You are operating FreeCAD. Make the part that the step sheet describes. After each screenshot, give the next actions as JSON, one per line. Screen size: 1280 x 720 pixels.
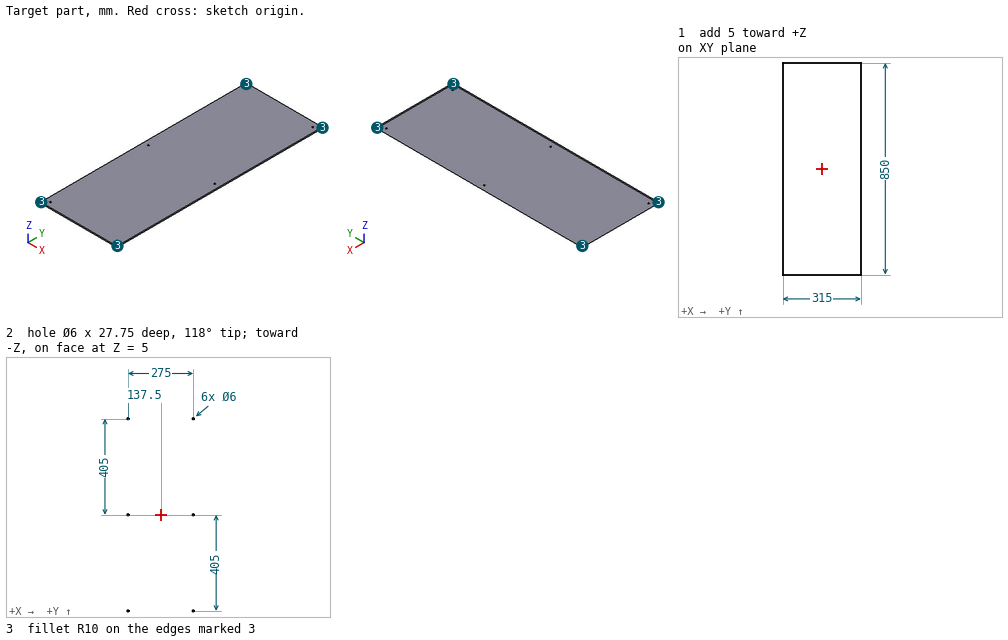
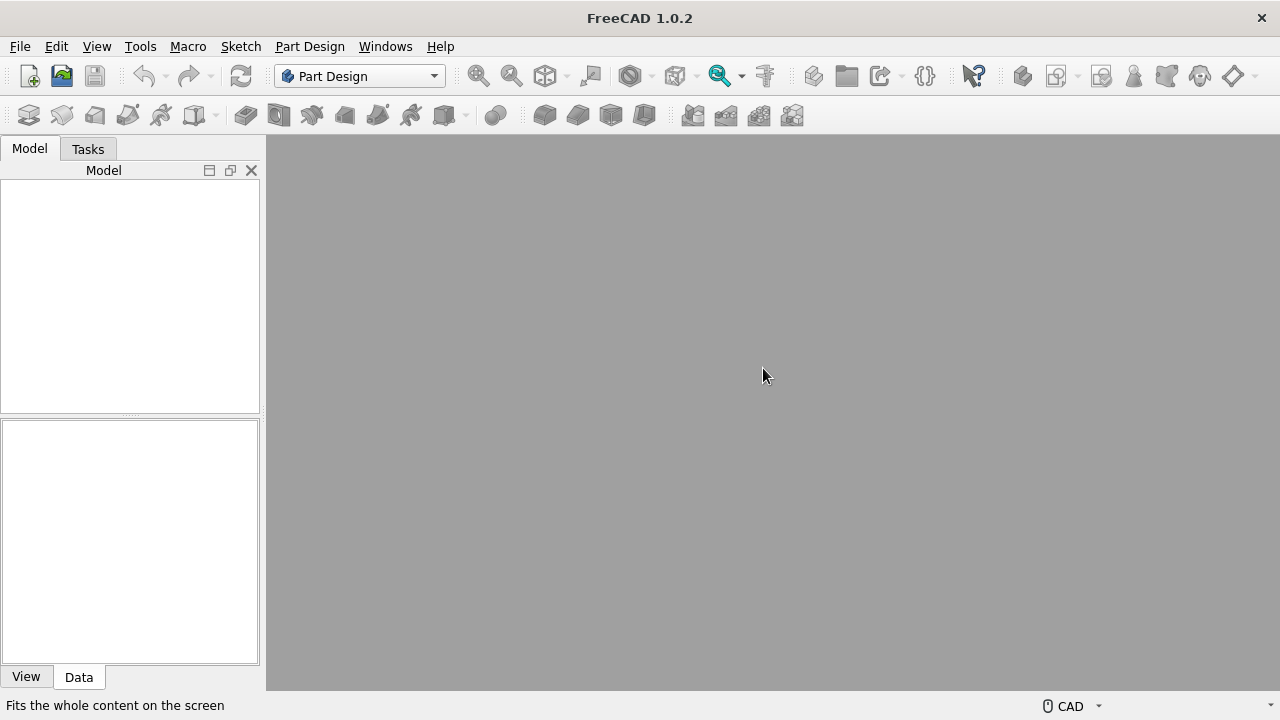
{"action": "left_click", "coordinate": [29, 76]}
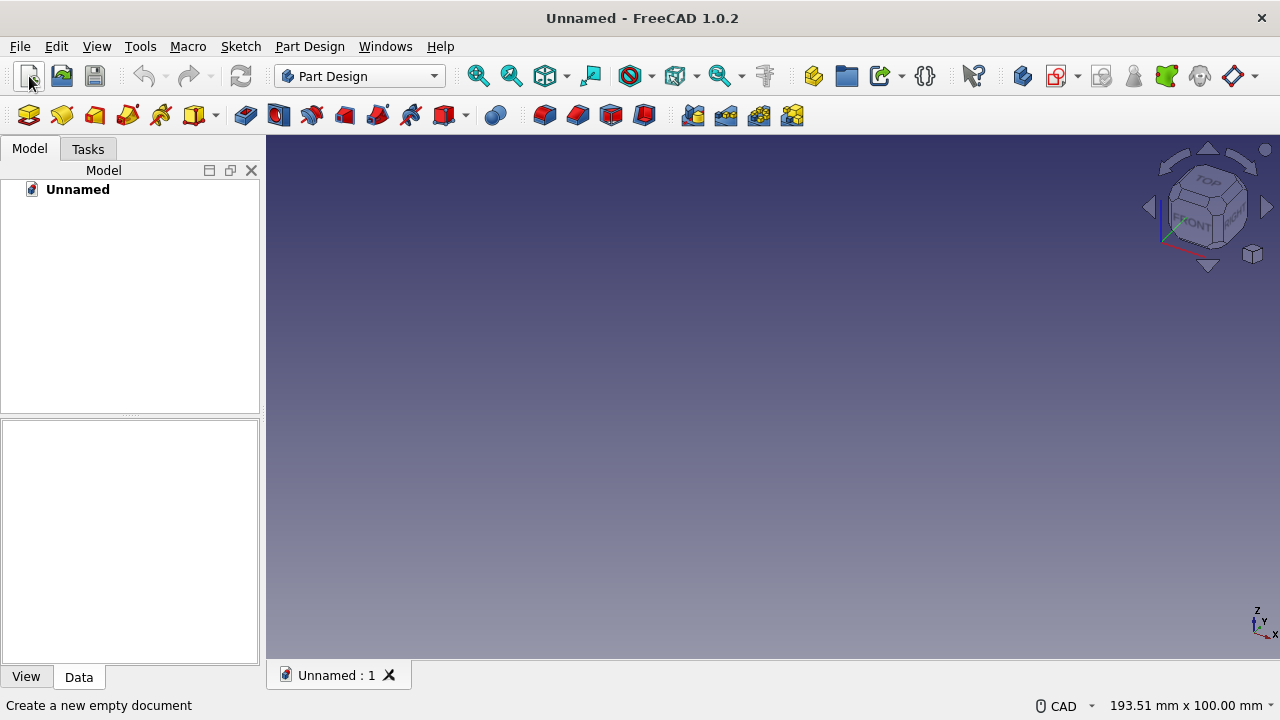
{"action": "left_click", "coordinate": [1056, 76]}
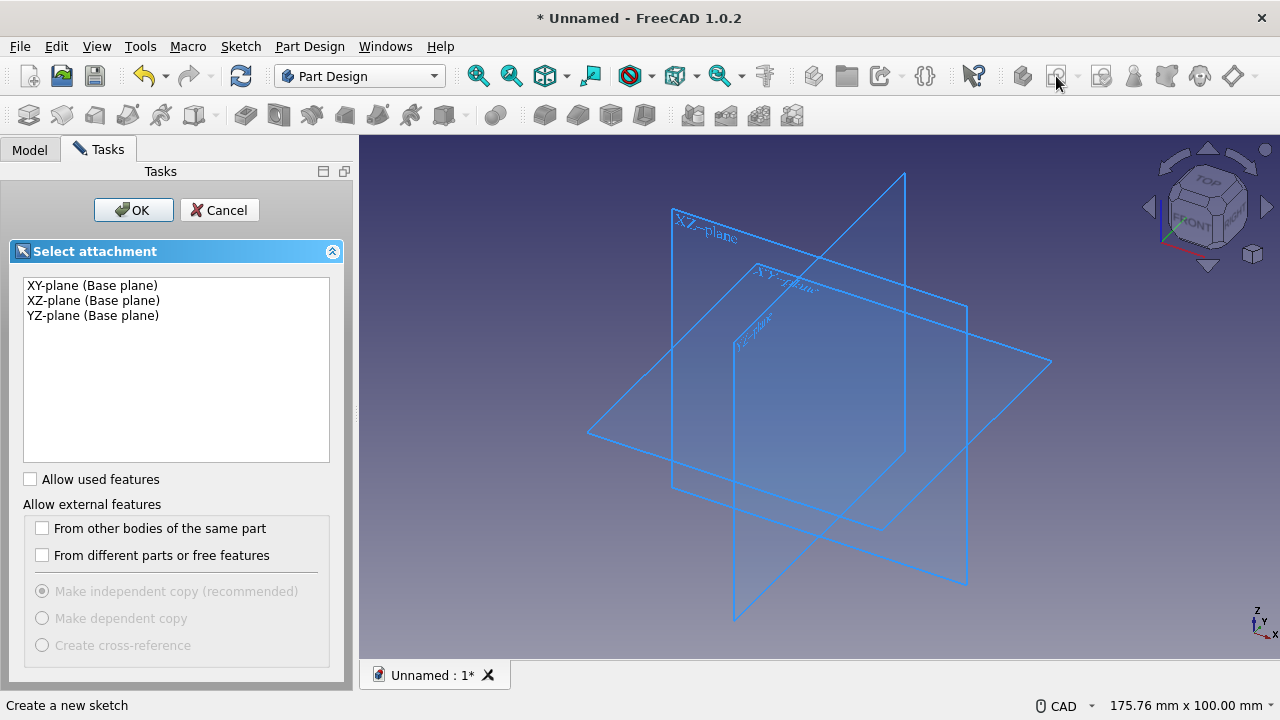
{"action": "left_click", "coordinate": [84, 286]}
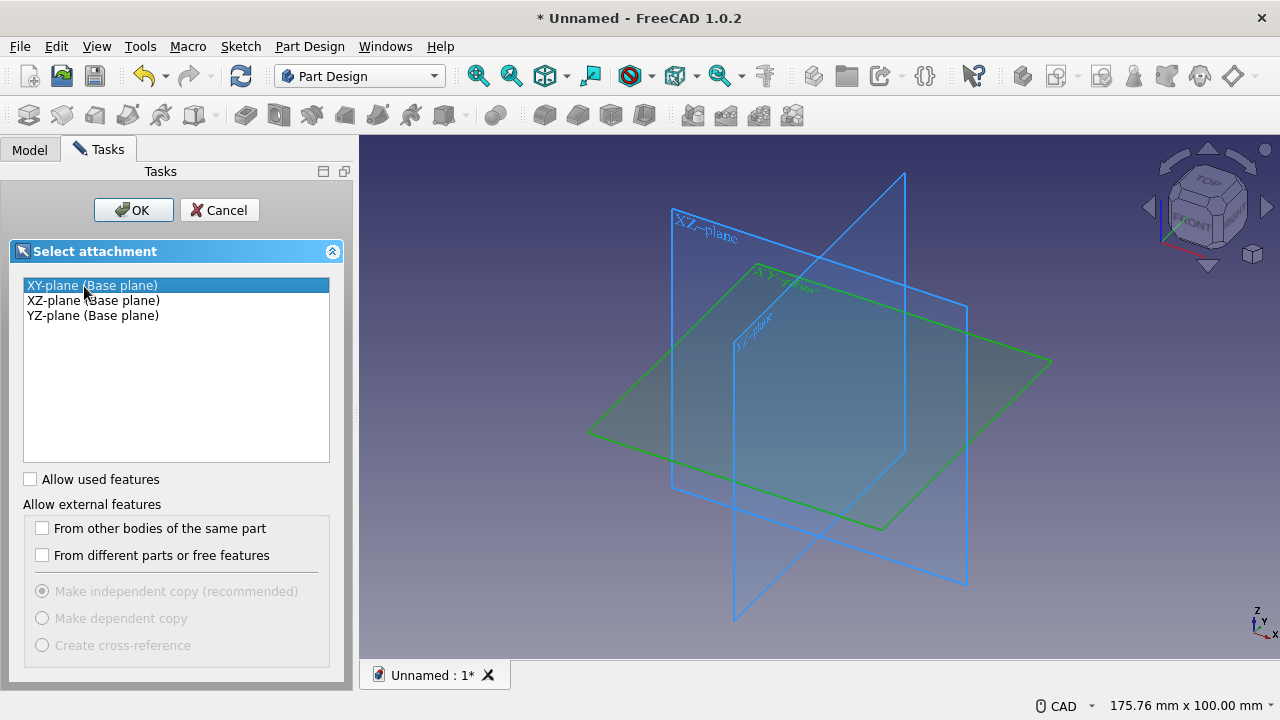
{"action": "left_click", "coordinate": [134, 210]}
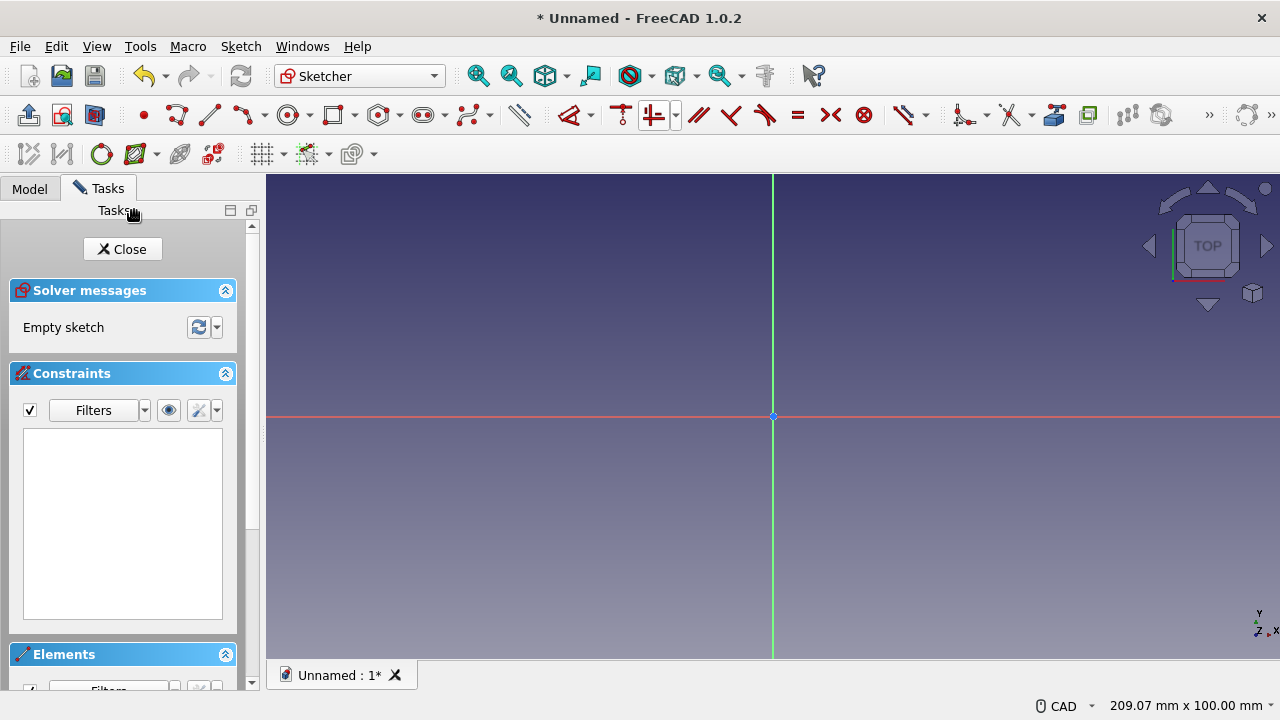
{"action": "scroll", "coordinate": [699, 416], "scroll_direction": "down", "scroll_amount": 13}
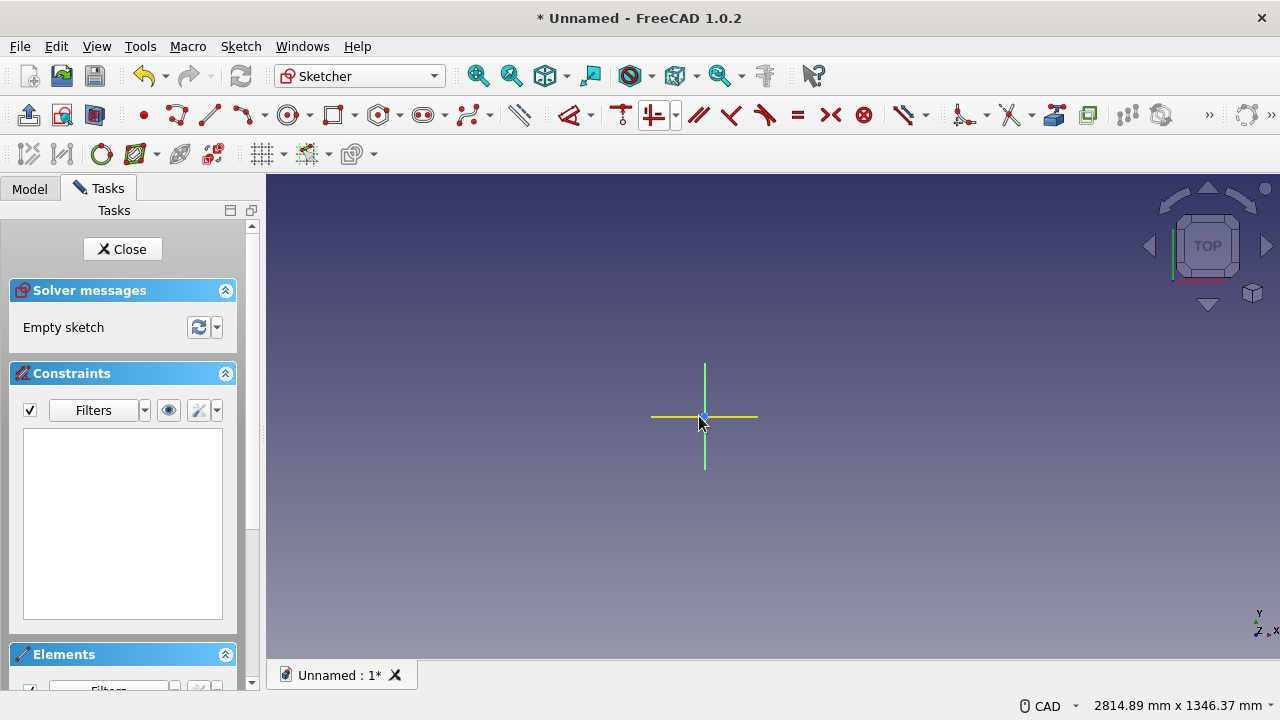
{"action": "left_click", "coordinate": [354, 116]}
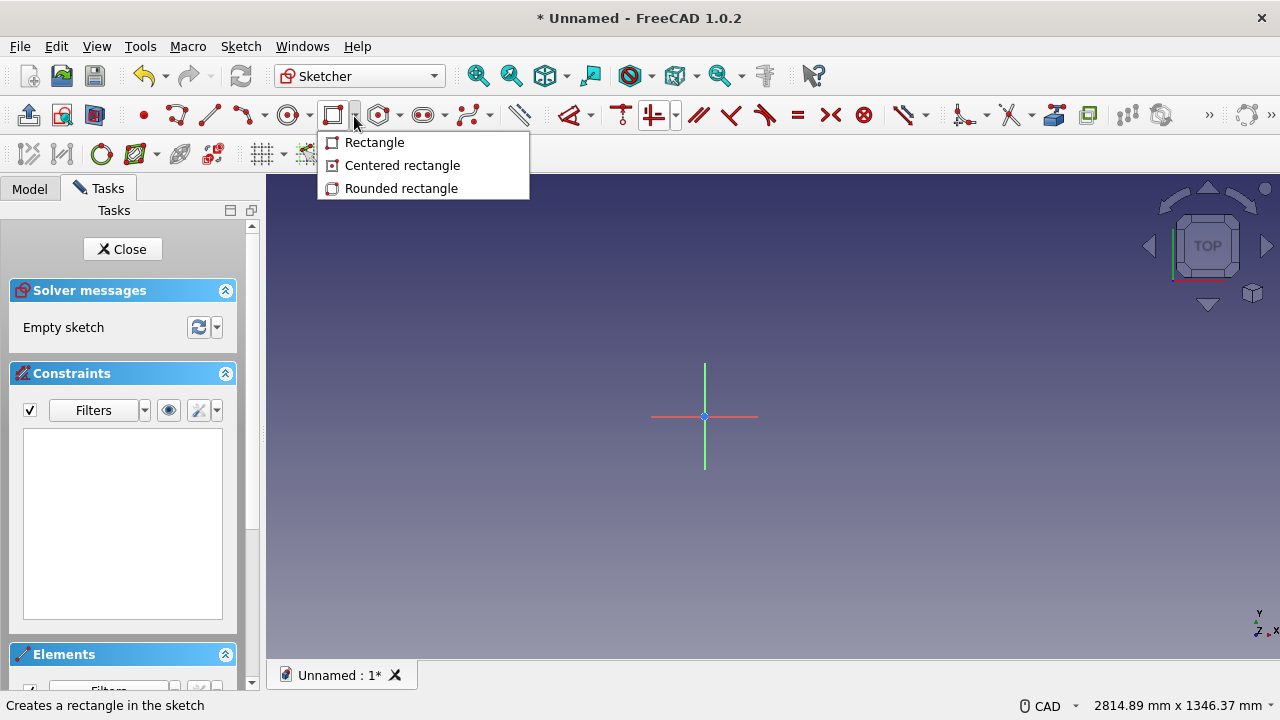
{"action": "left_click", "coordinate": [424, 166]}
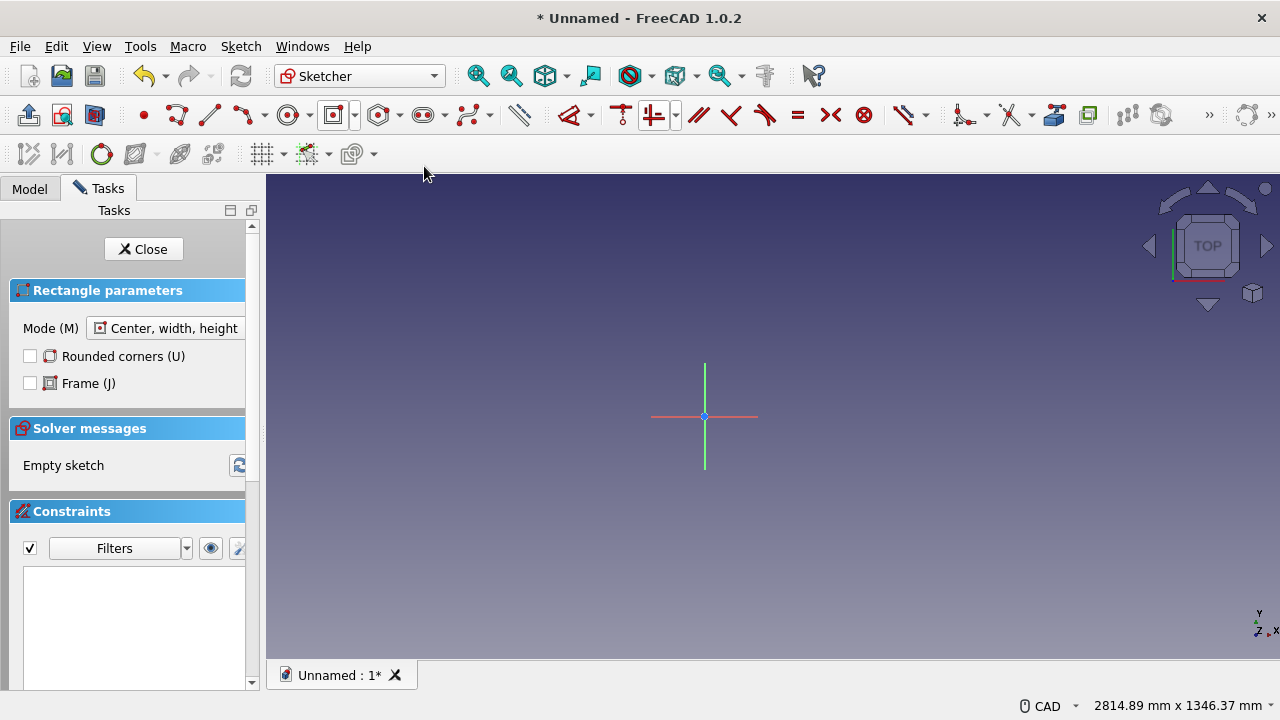
{"action": "left_click", "coordinate": [705, 416]}
{"action": "mouse_move", "coordinate": [762, 263]}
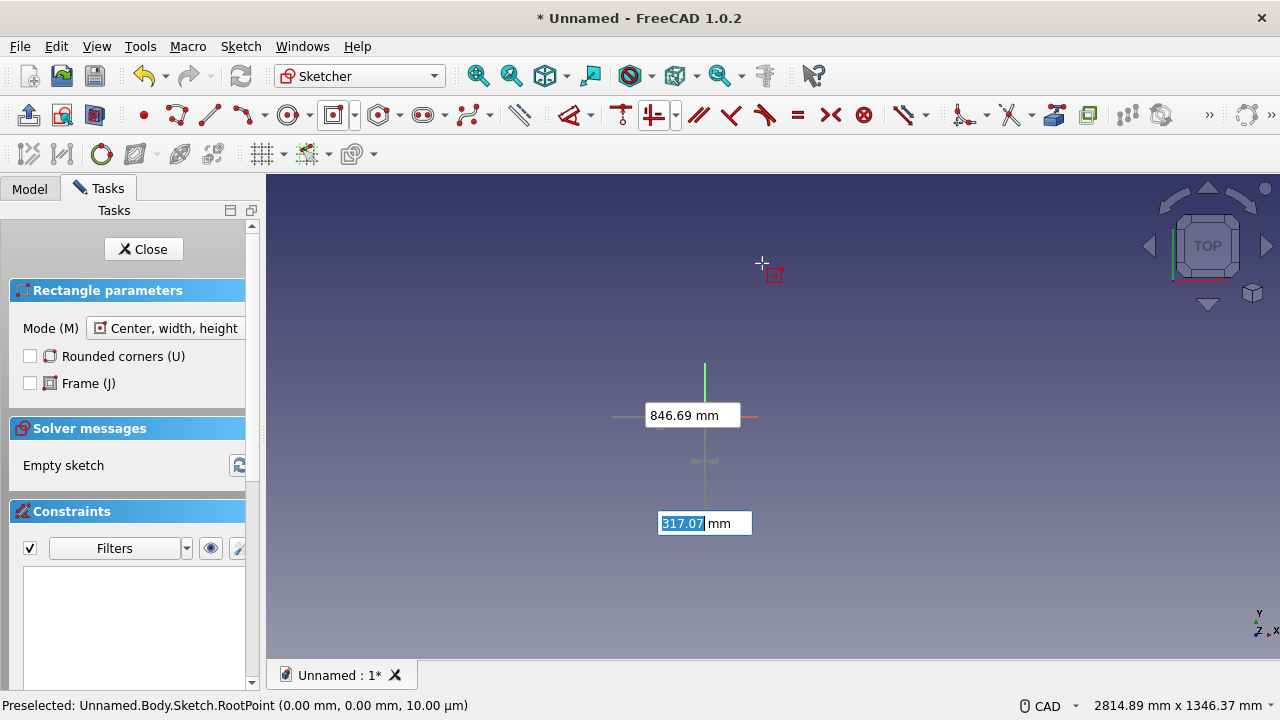
{"action": "type", "text": "315"}
{"action": "key", "text": "Tab"}
{"action": "type", "text": "850"}
{"action": "key", "text": "Return"}
{"action": "key", "text": "Escape"}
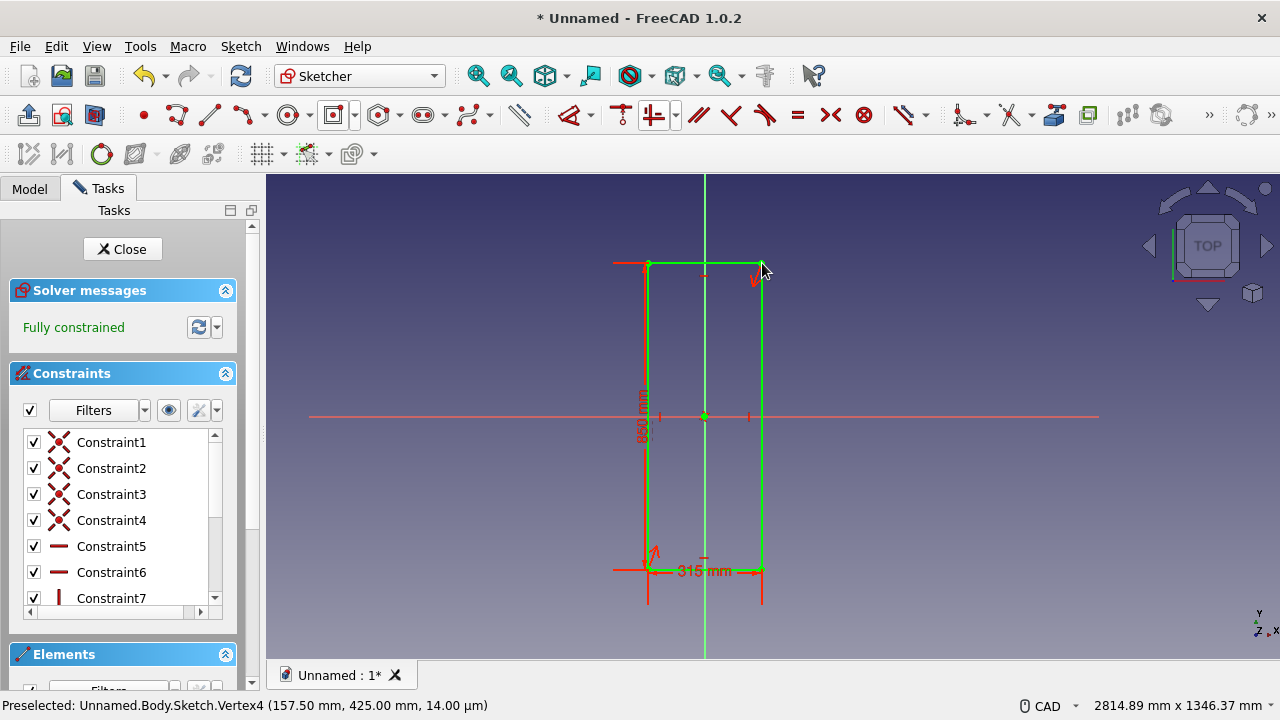
{"action": "left_click", "coordinate": [123, 249]}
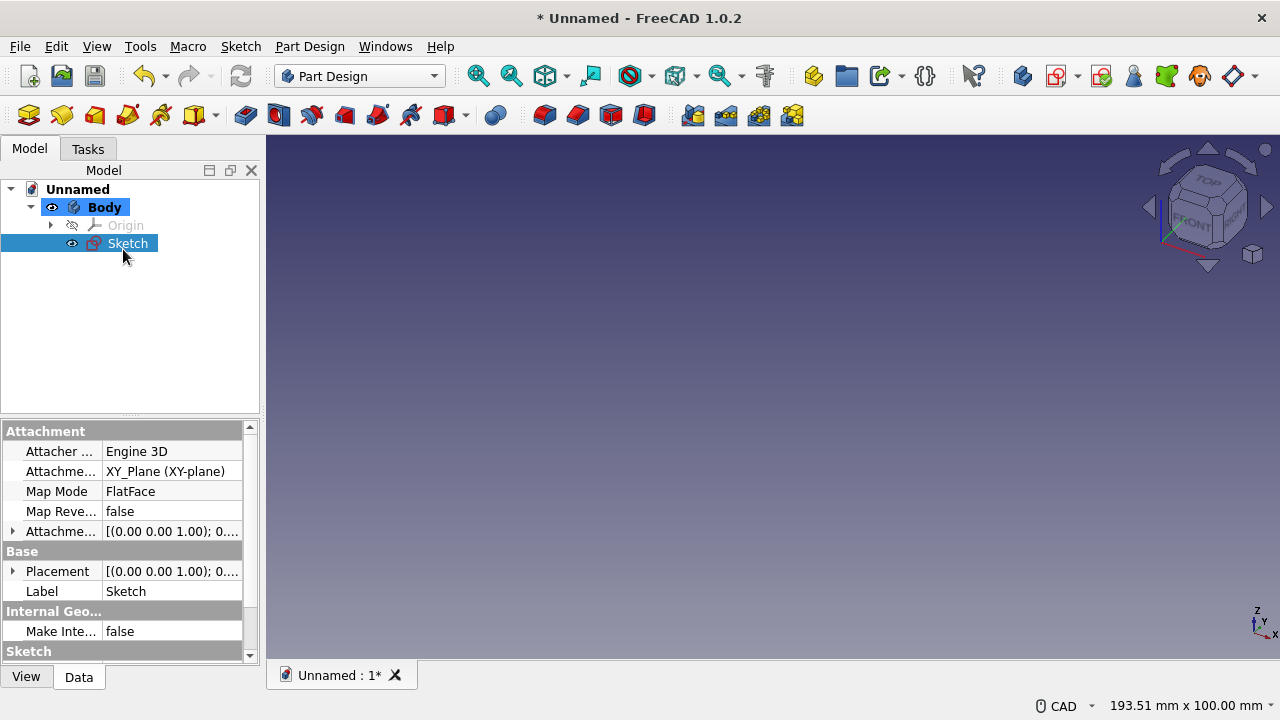
{"action": "left_click", "coordinate": [29, 116]}